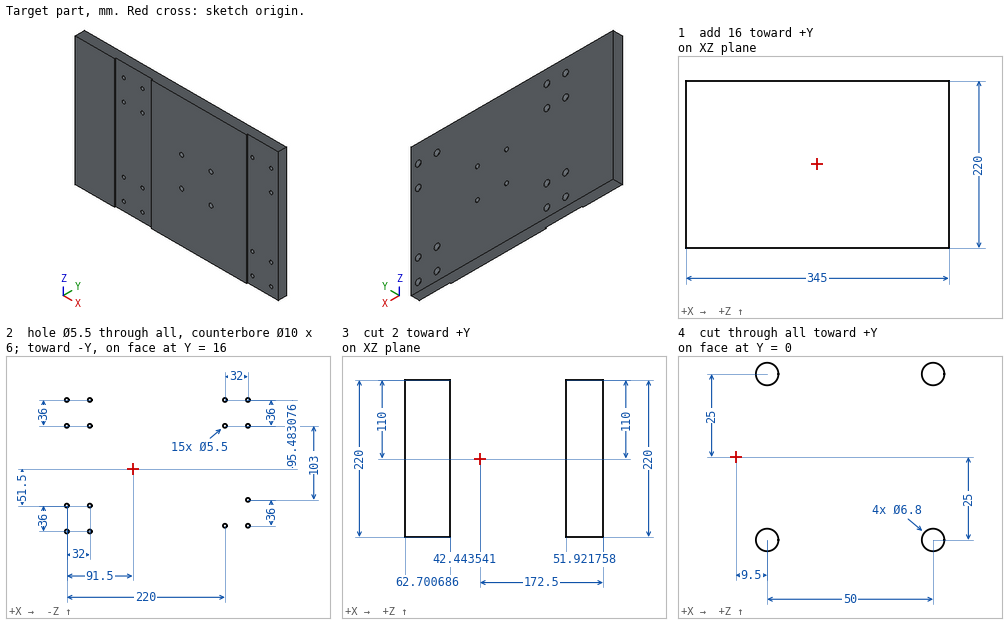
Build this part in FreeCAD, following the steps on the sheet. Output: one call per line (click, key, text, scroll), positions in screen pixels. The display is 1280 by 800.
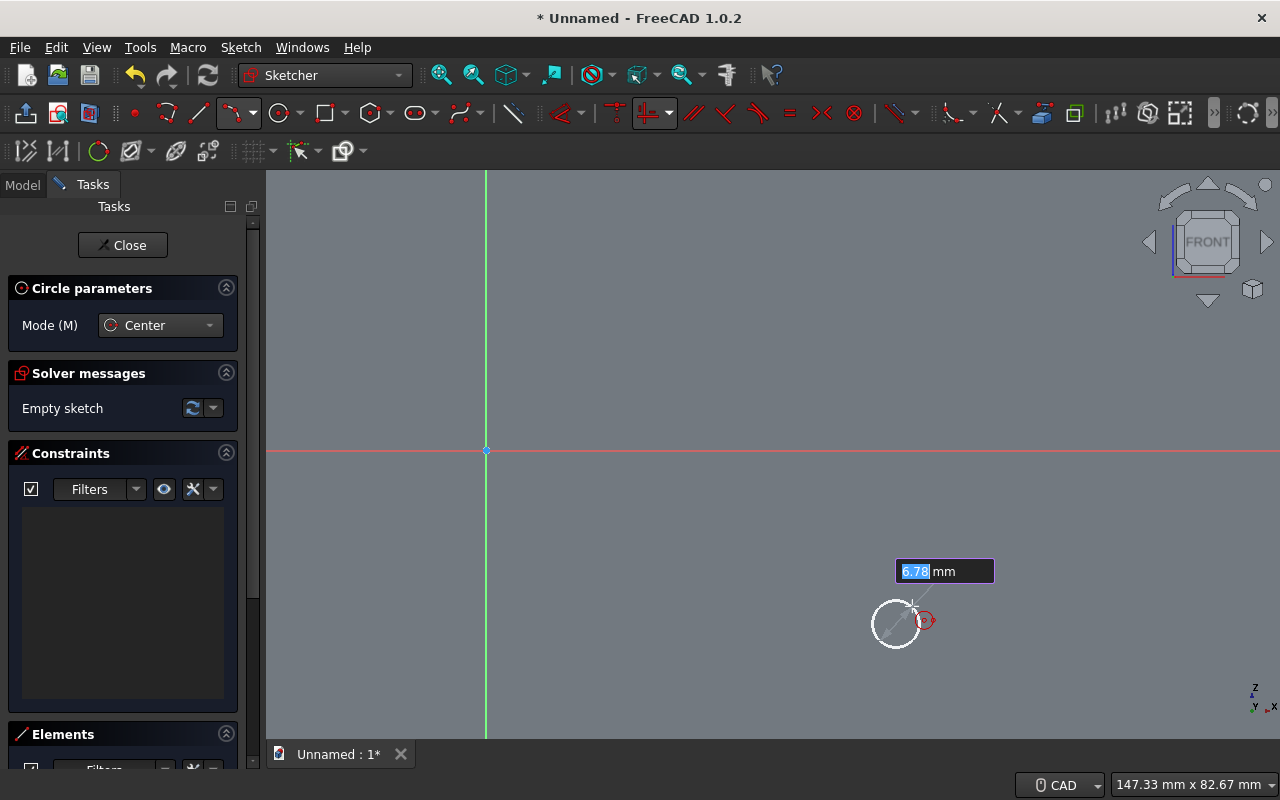
text(6.8)
key(Return)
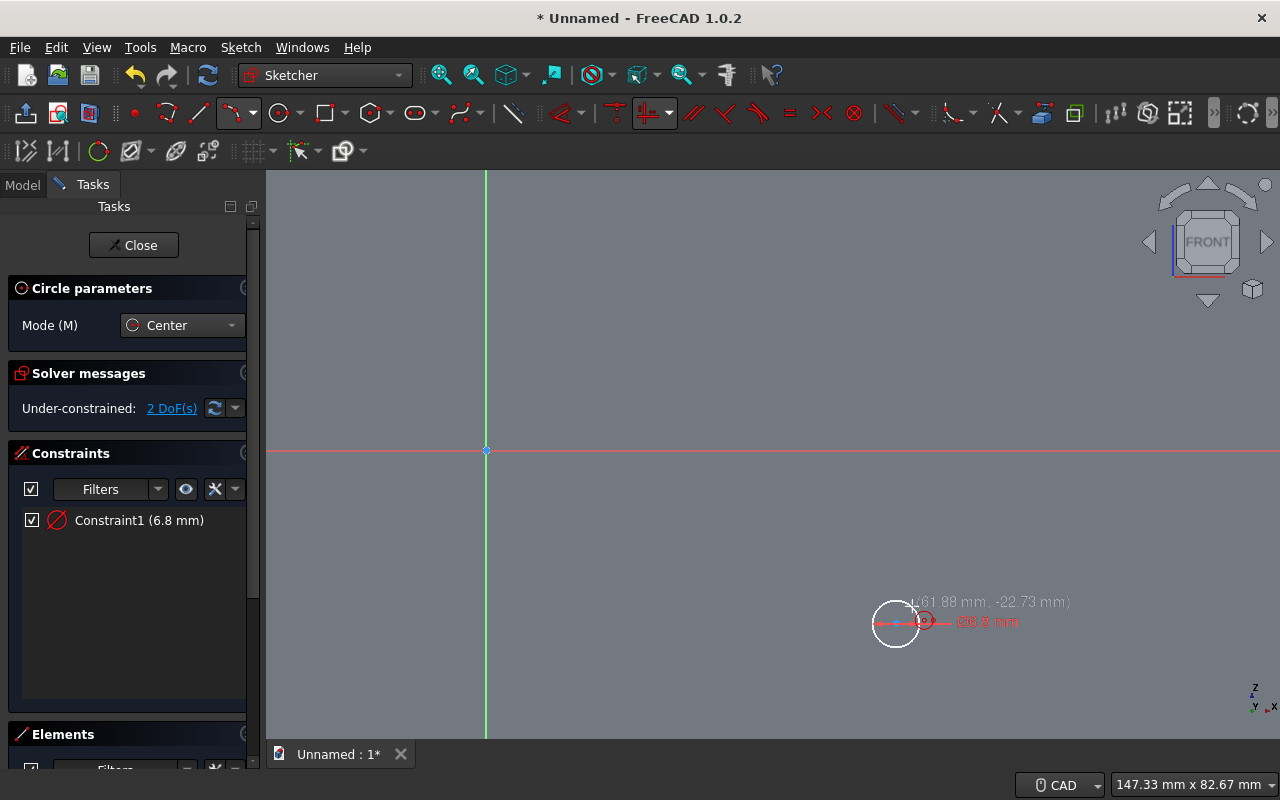
click(552, 623)
move(568, 606)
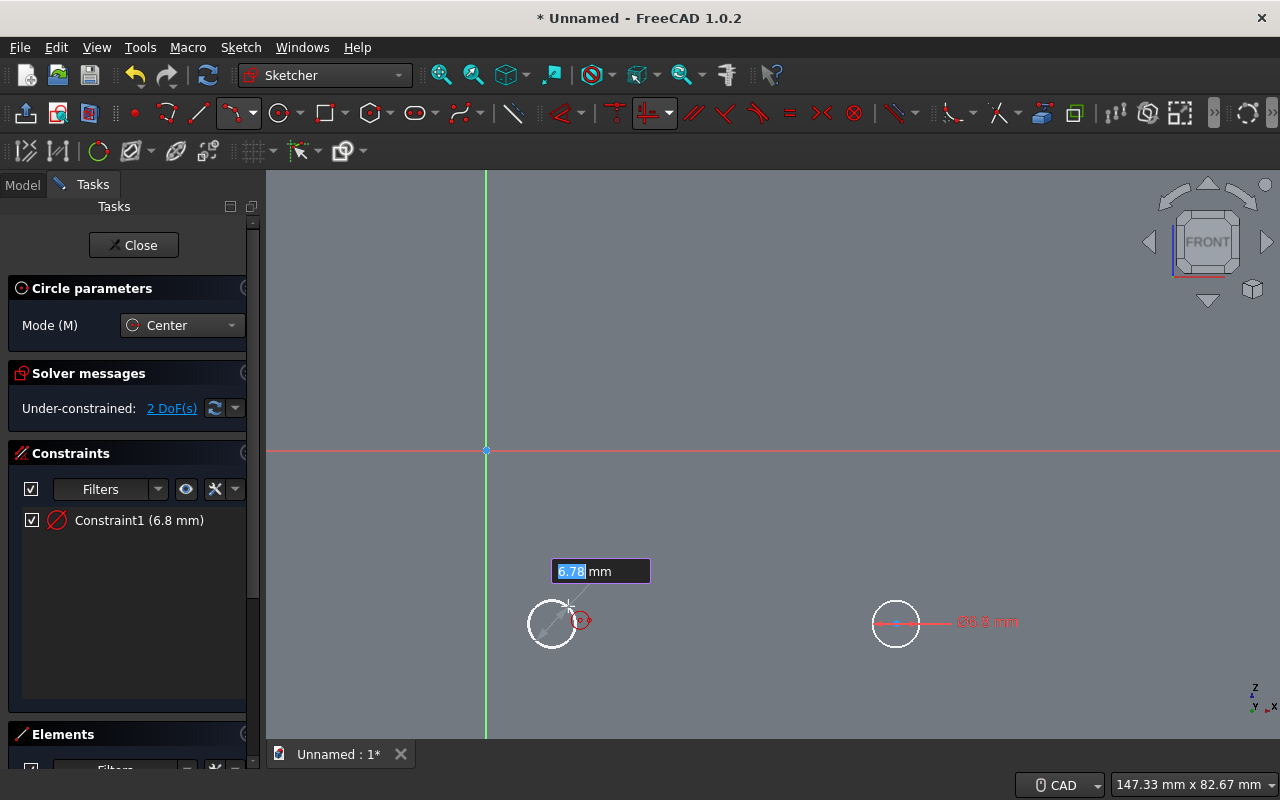
text(6.8)
key(Return)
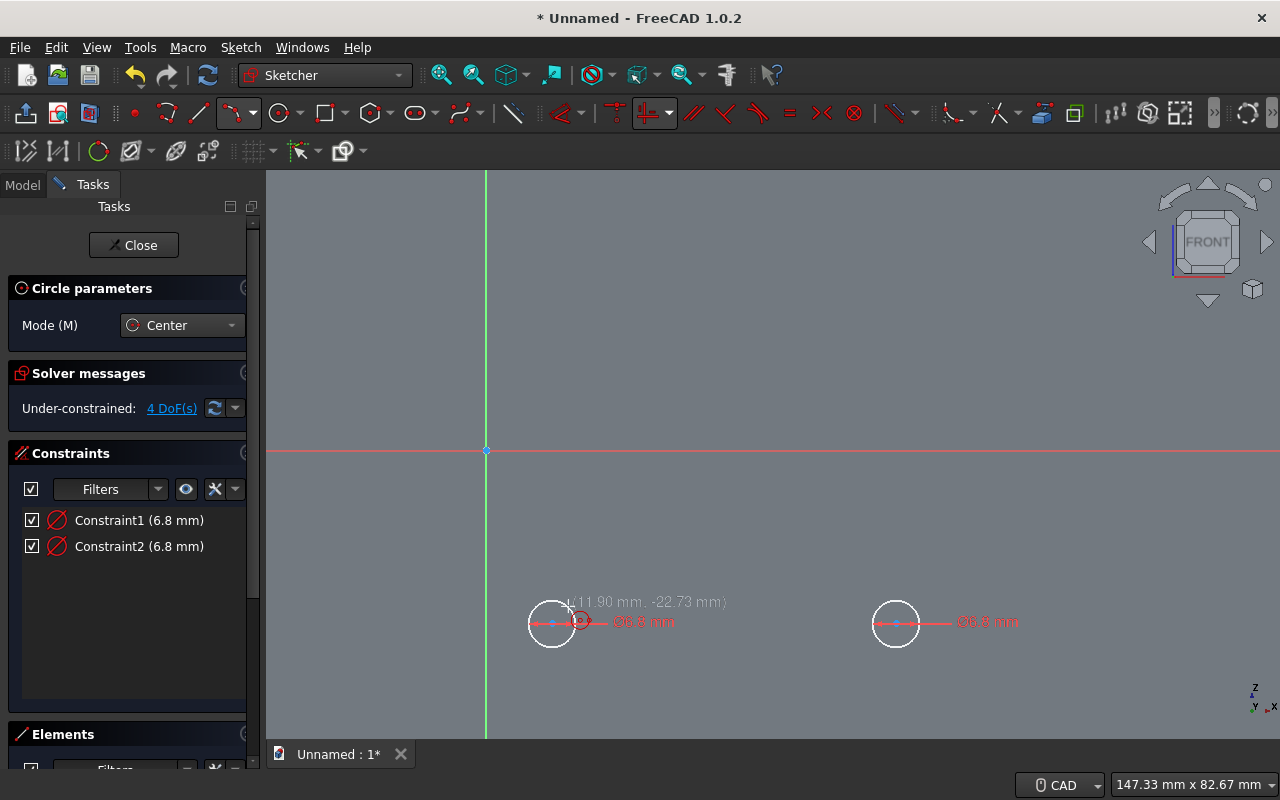
click(552, 278)
move(568, 262)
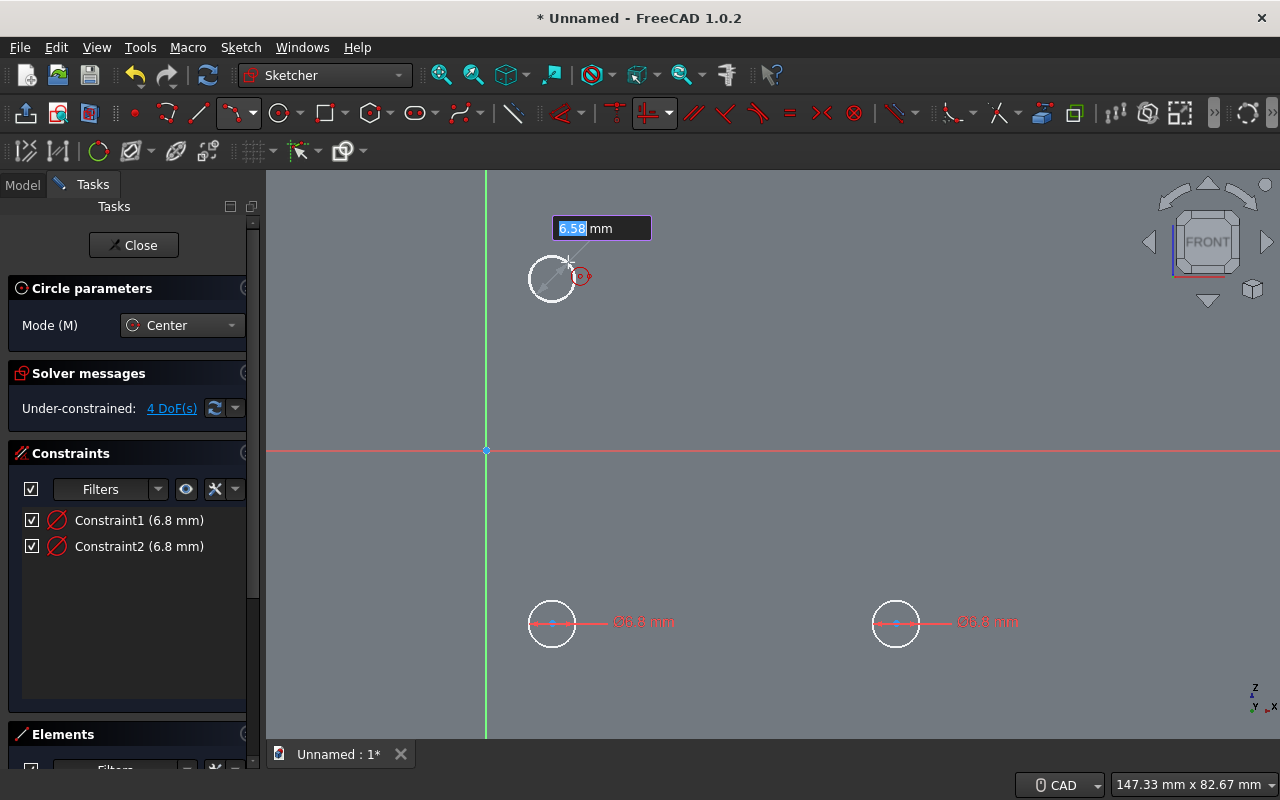
text(6.8)
key(Return)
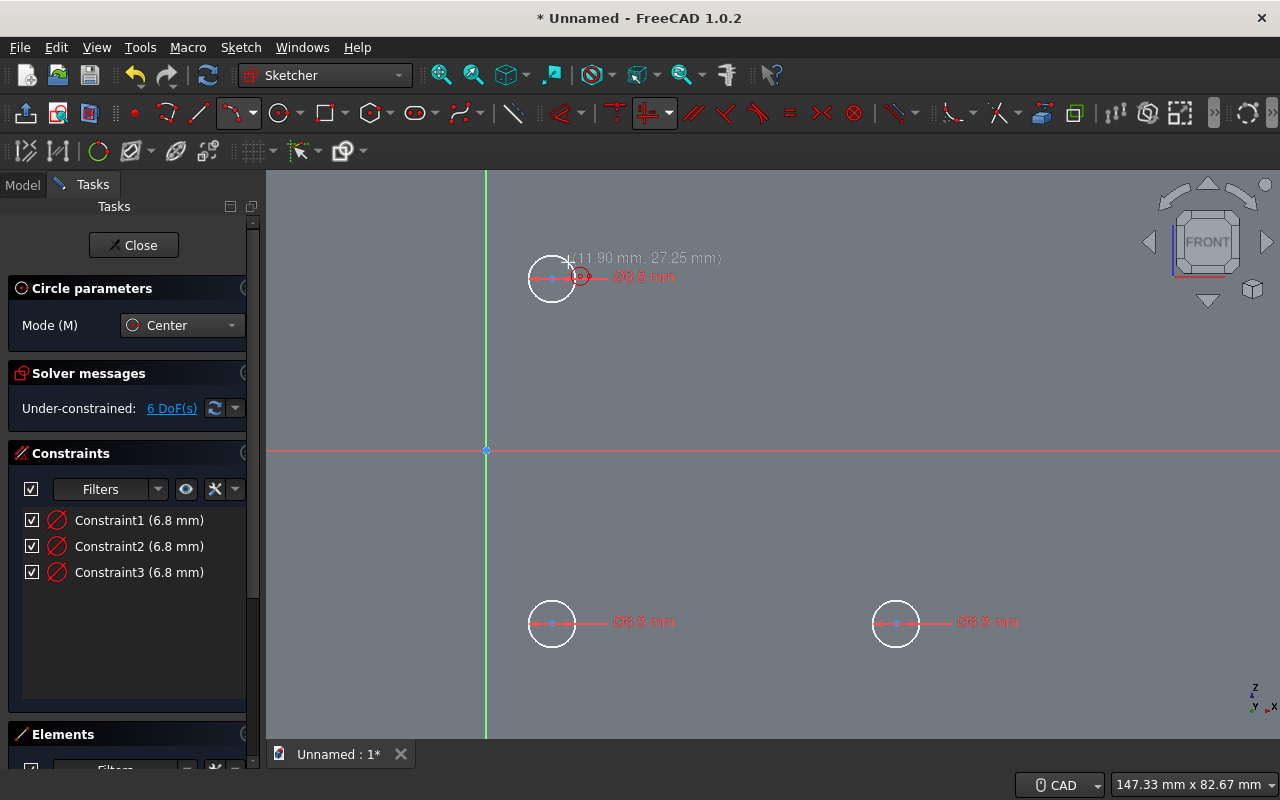
click(896, 278)
move(912, 262)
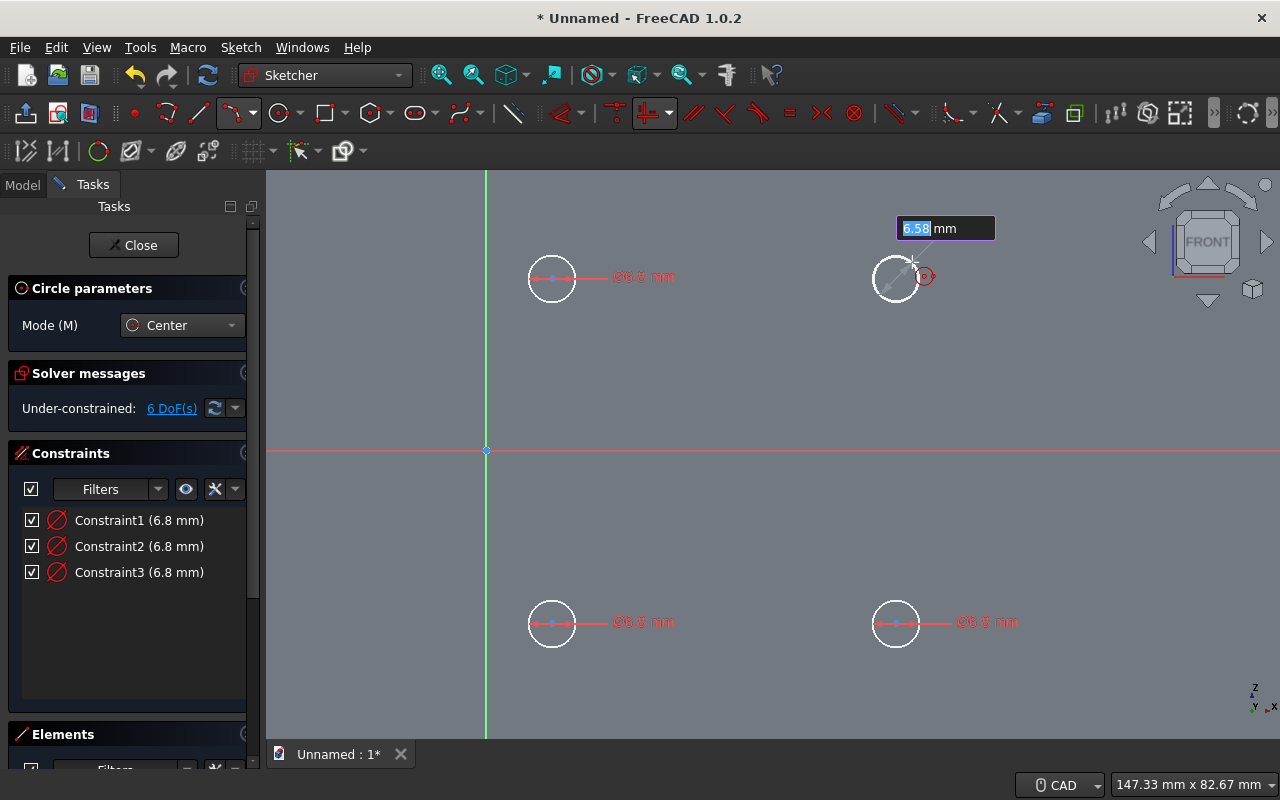
text(6.8)
key(Return)
key(Escape)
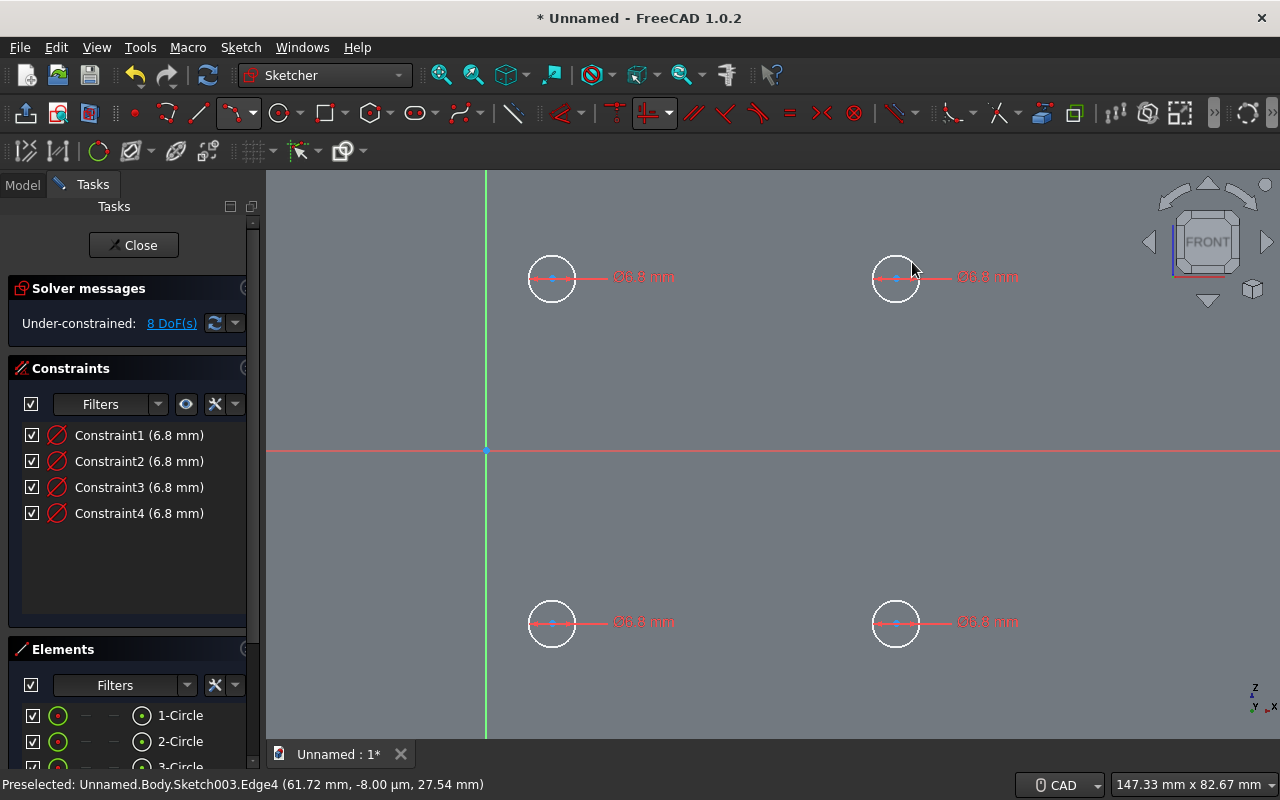
click(896, 624)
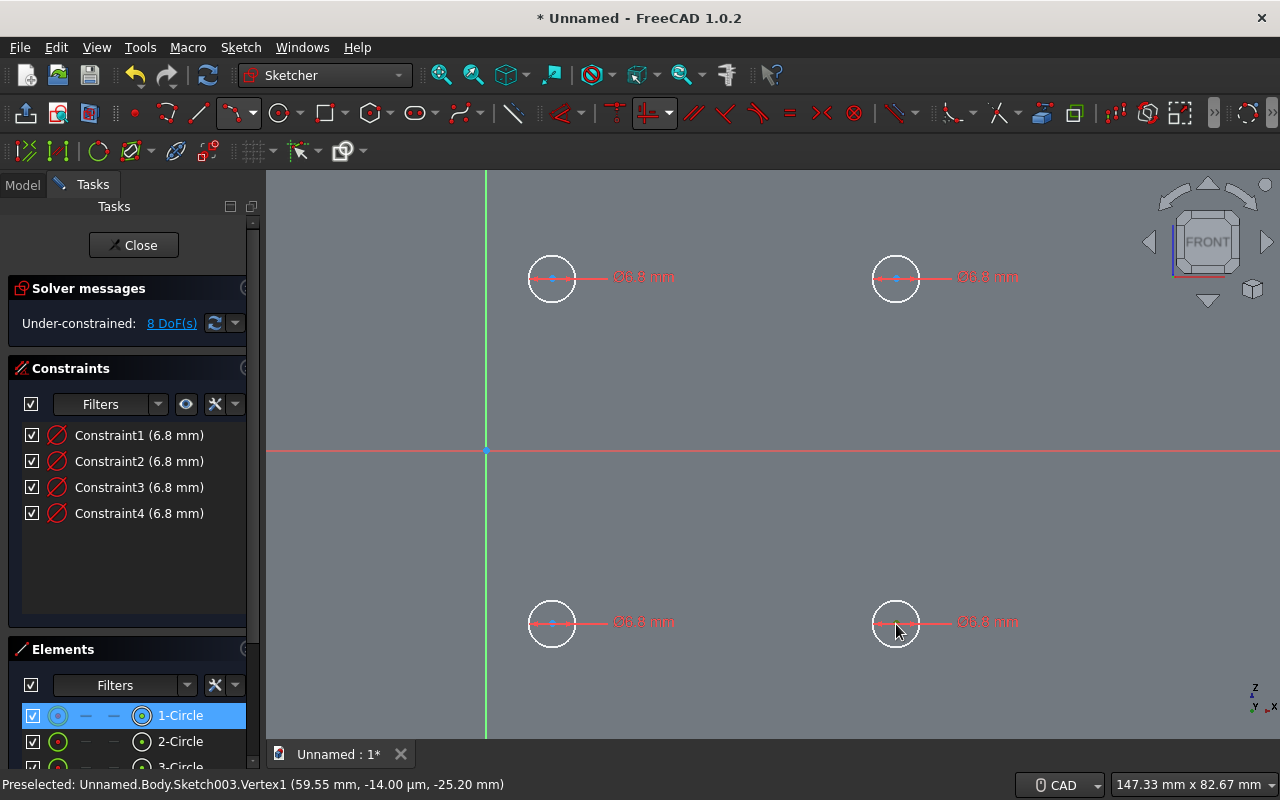
click(552, 624)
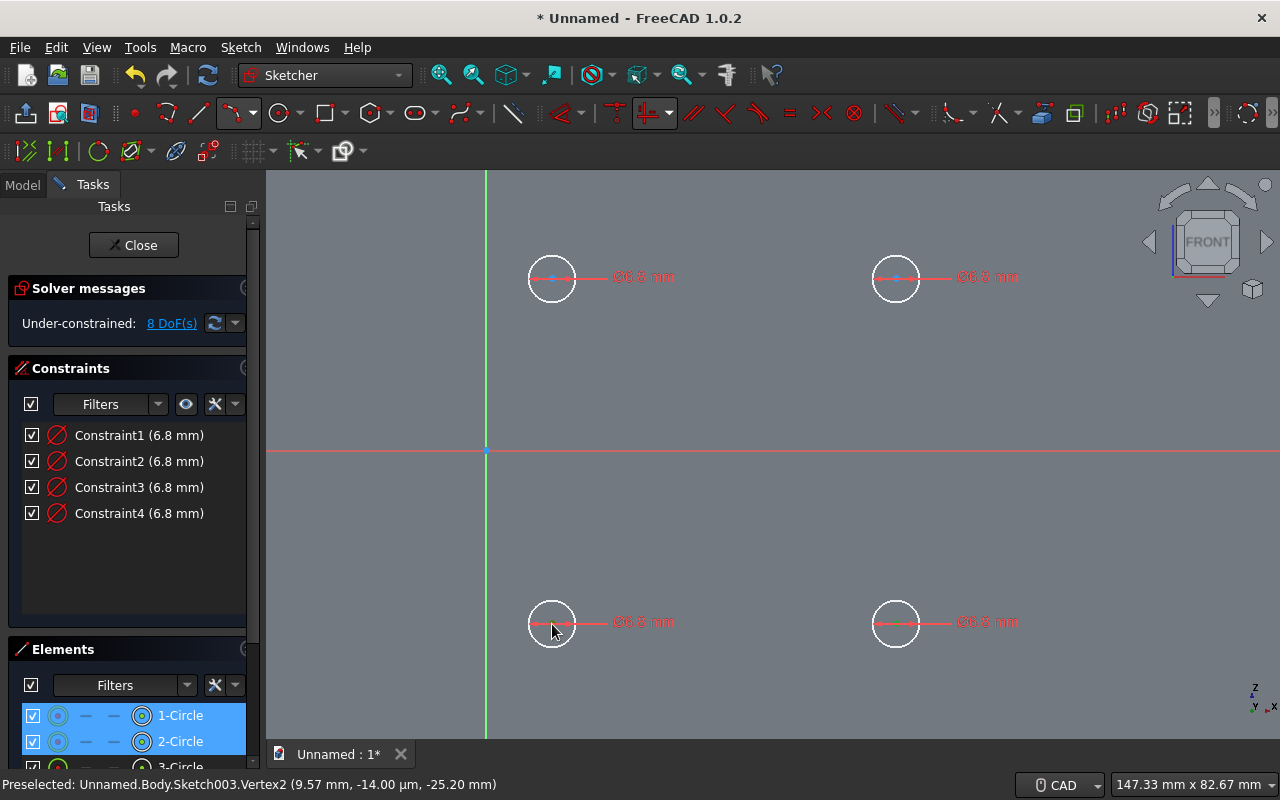
key(h)